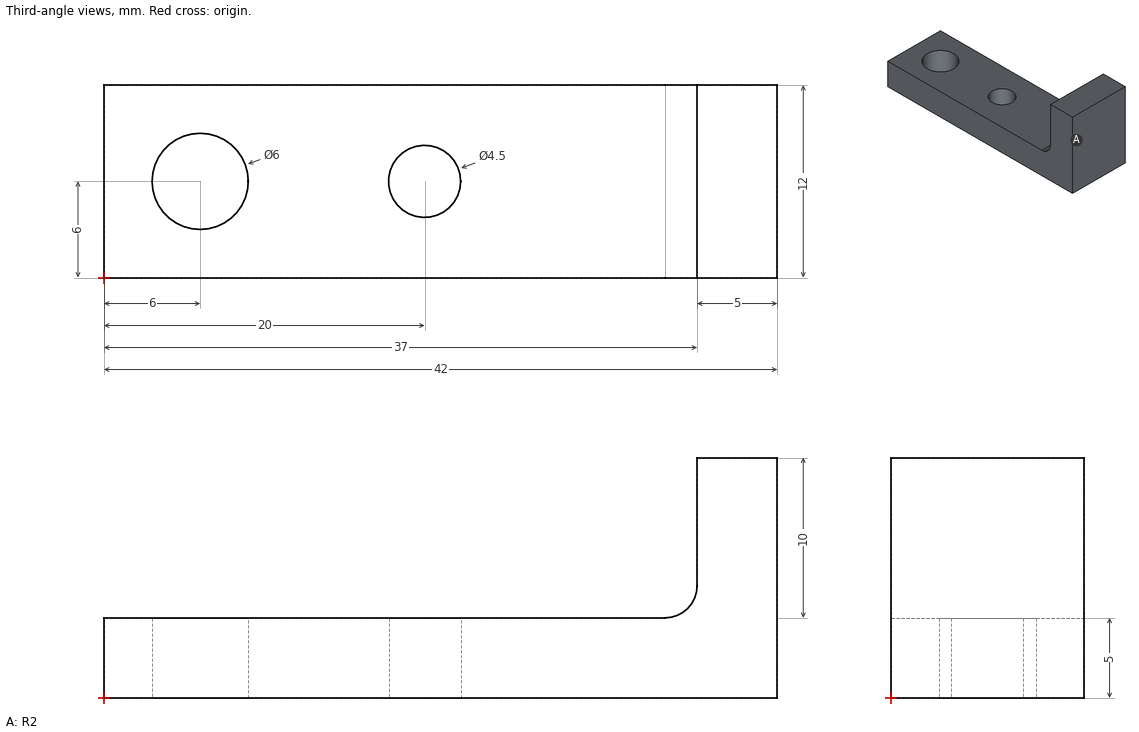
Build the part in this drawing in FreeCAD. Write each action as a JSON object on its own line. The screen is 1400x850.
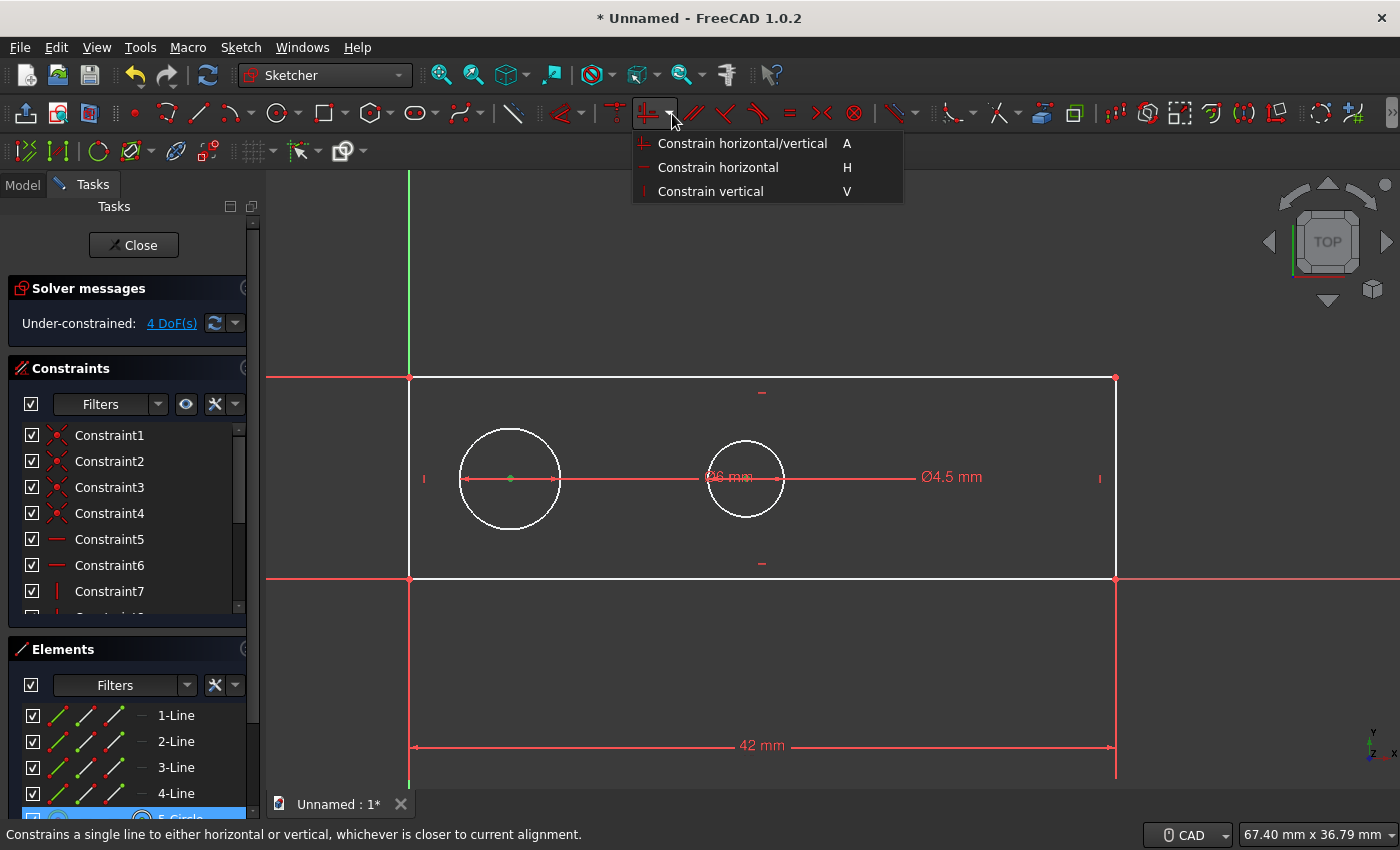
{"action": "left_click", "coordinate": [768, 167]}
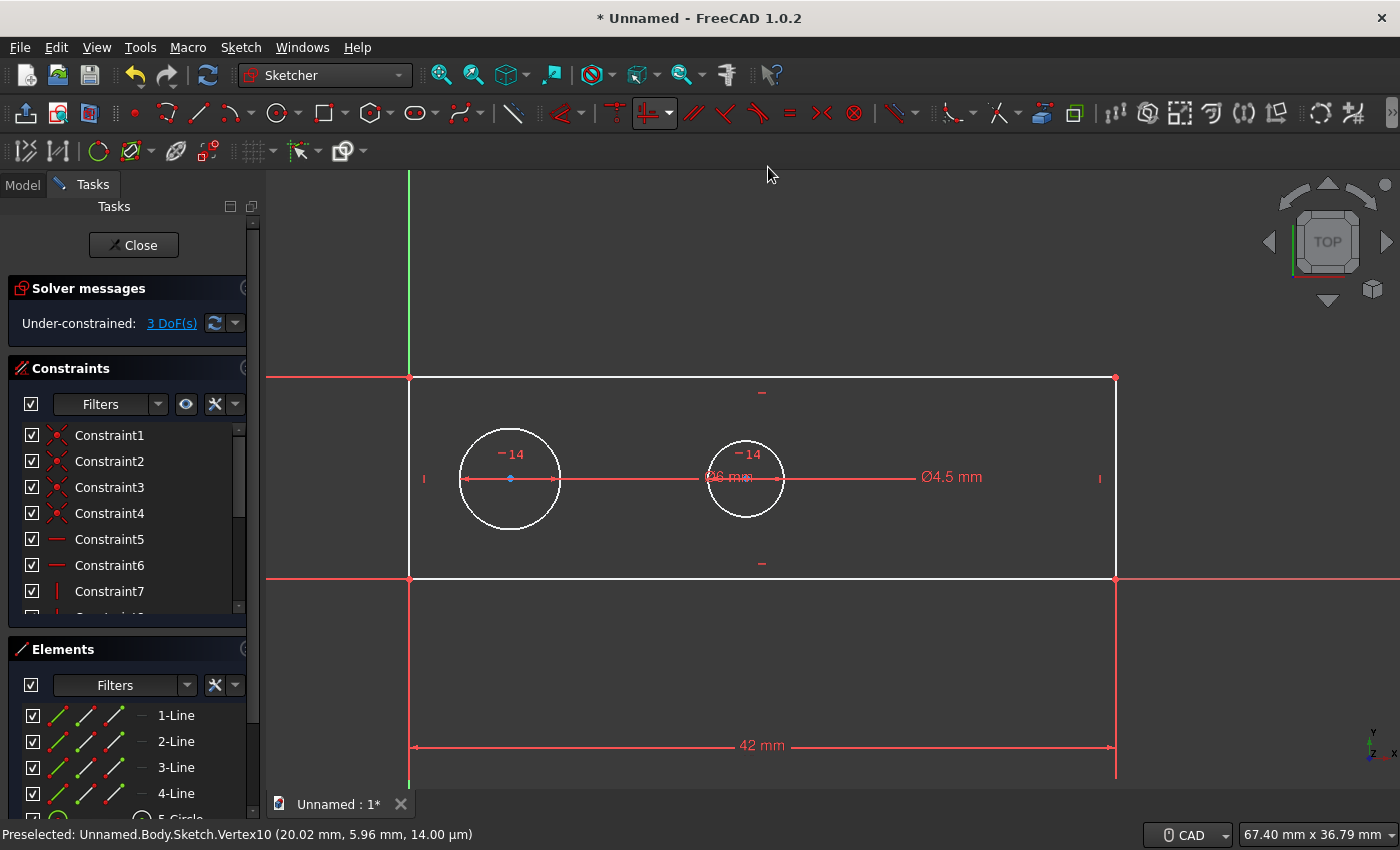
{"action": "key", "text": "d"}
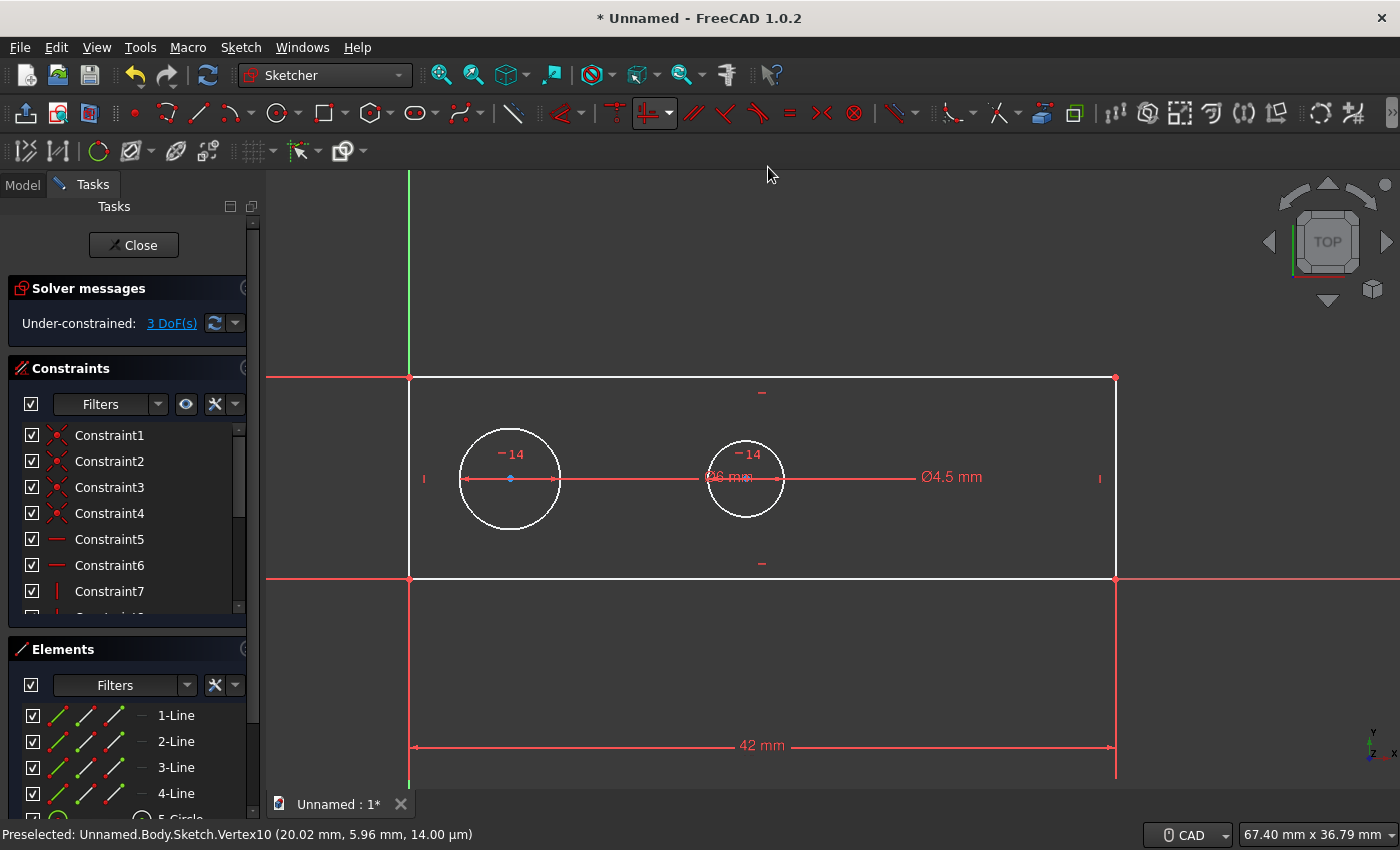
{"action": "left_click", "coordinate": [510, 479]}
{"action": "left_click", "coordinate": [460, 613]}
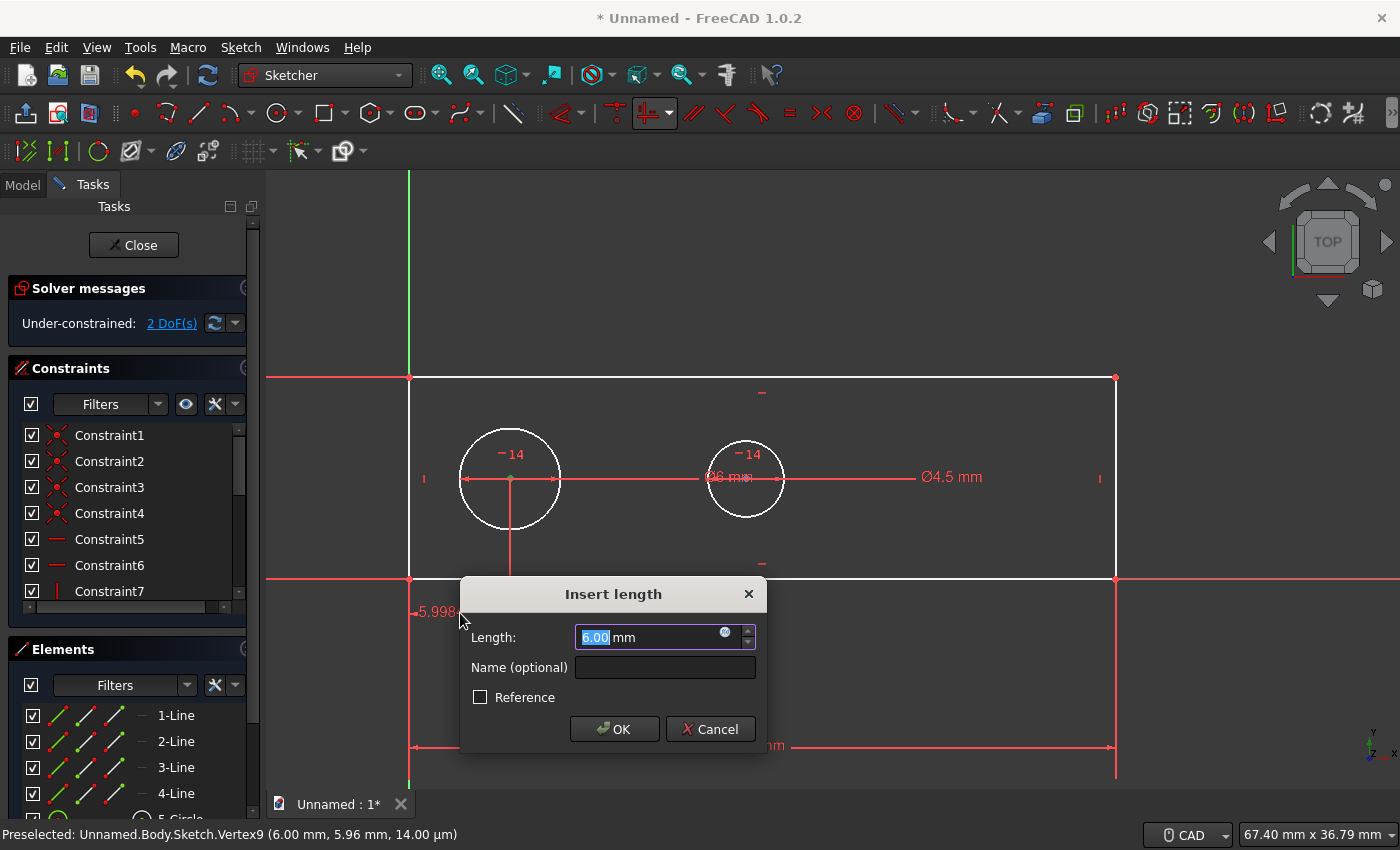
{"action": "type", "text": "6"}
{"action": "key", "text": "Return"}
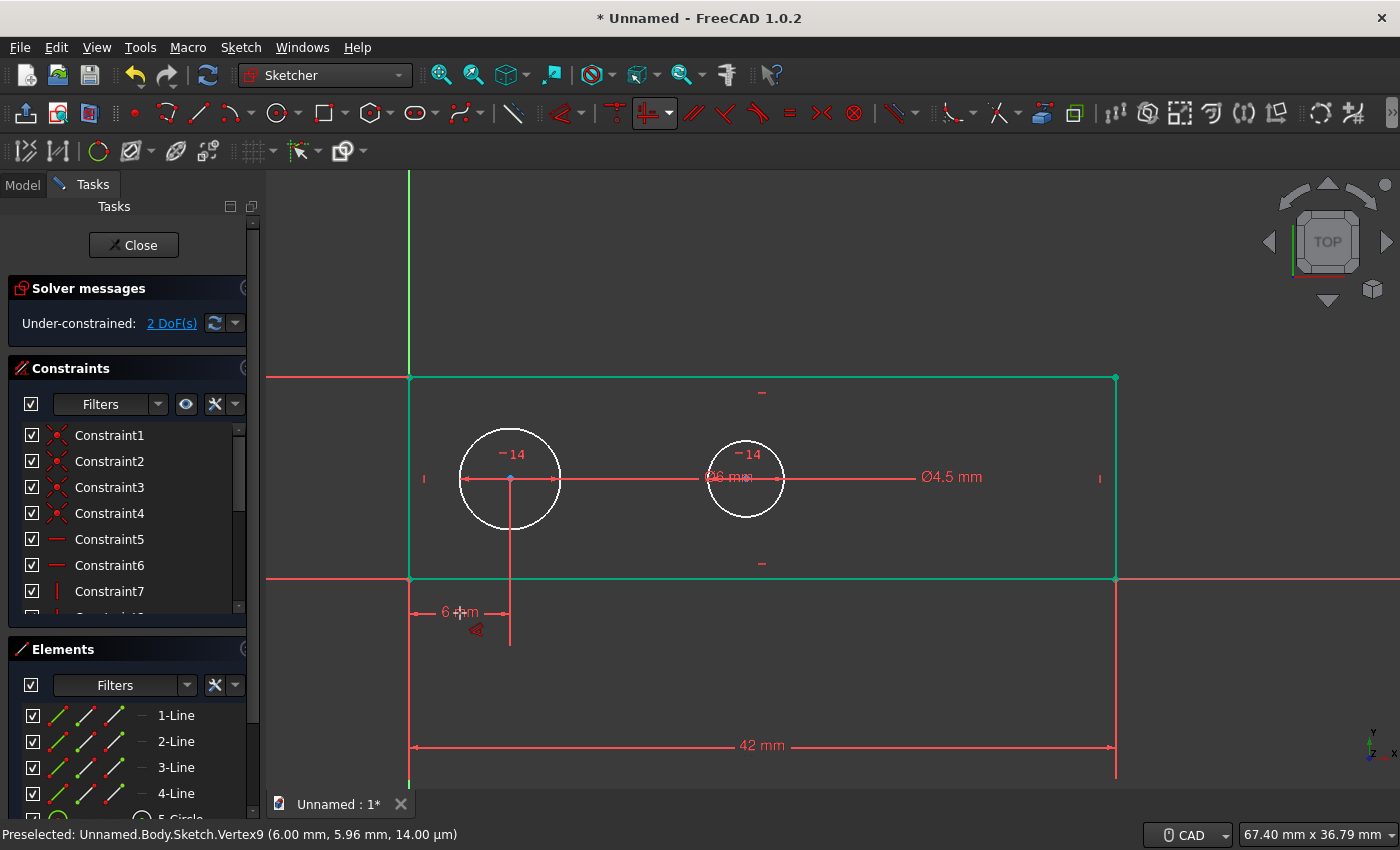
{"action": "left_click", "coordinate": [510, 479]}
{"action": "left_click", "coordinate": [375, 529]}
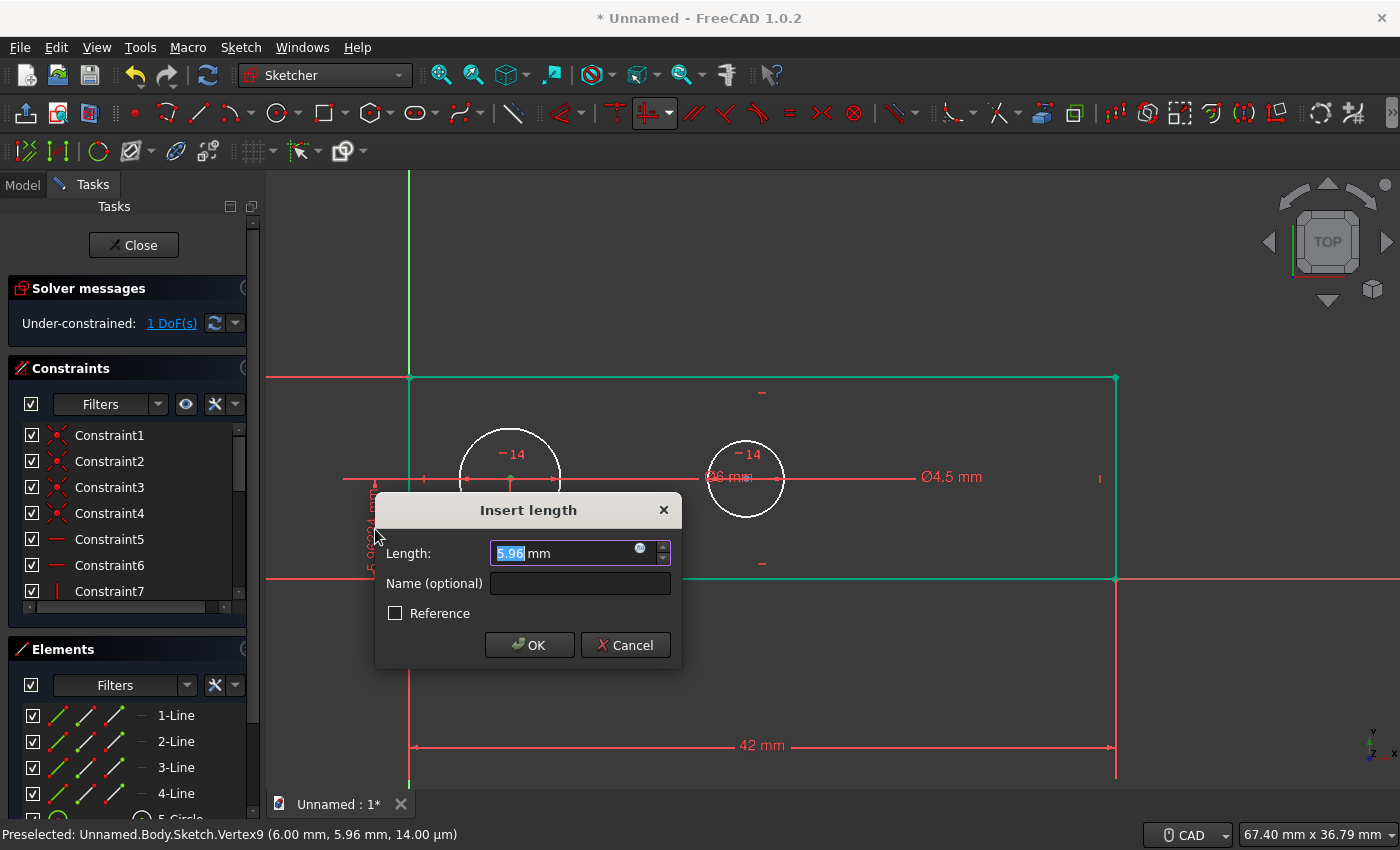
{"action": "type", "text": "6"}
{"action": "key", "text": "Return"}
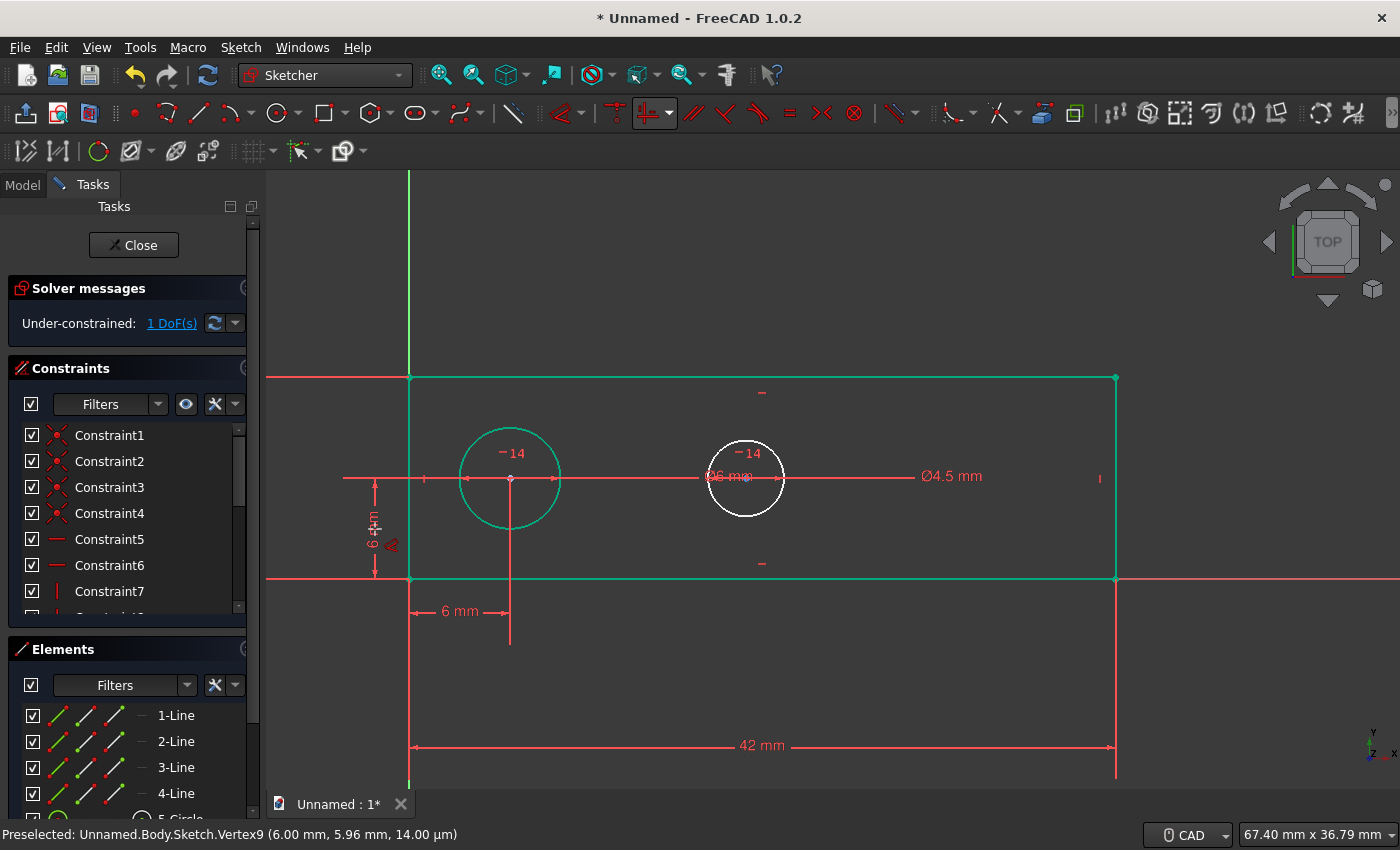
{"action": "left_click", "coordinate": [746, 478]}
{"action": "left_click", "coordinate": [578, 613]}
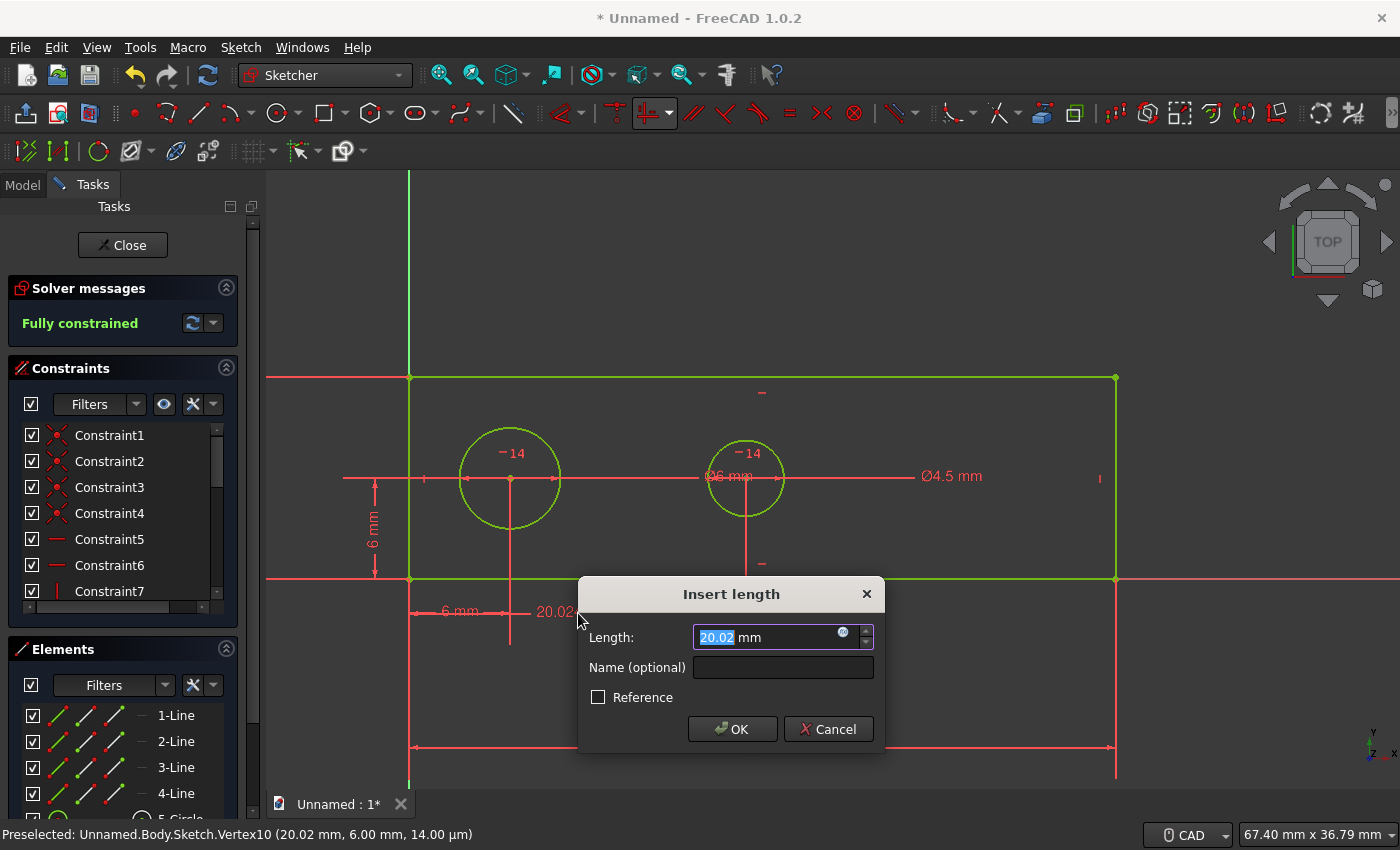
{"action": "type", "text": "20"}
{"action": "key", "text": "Return"}
{"action": "key", "text": "Escape"}